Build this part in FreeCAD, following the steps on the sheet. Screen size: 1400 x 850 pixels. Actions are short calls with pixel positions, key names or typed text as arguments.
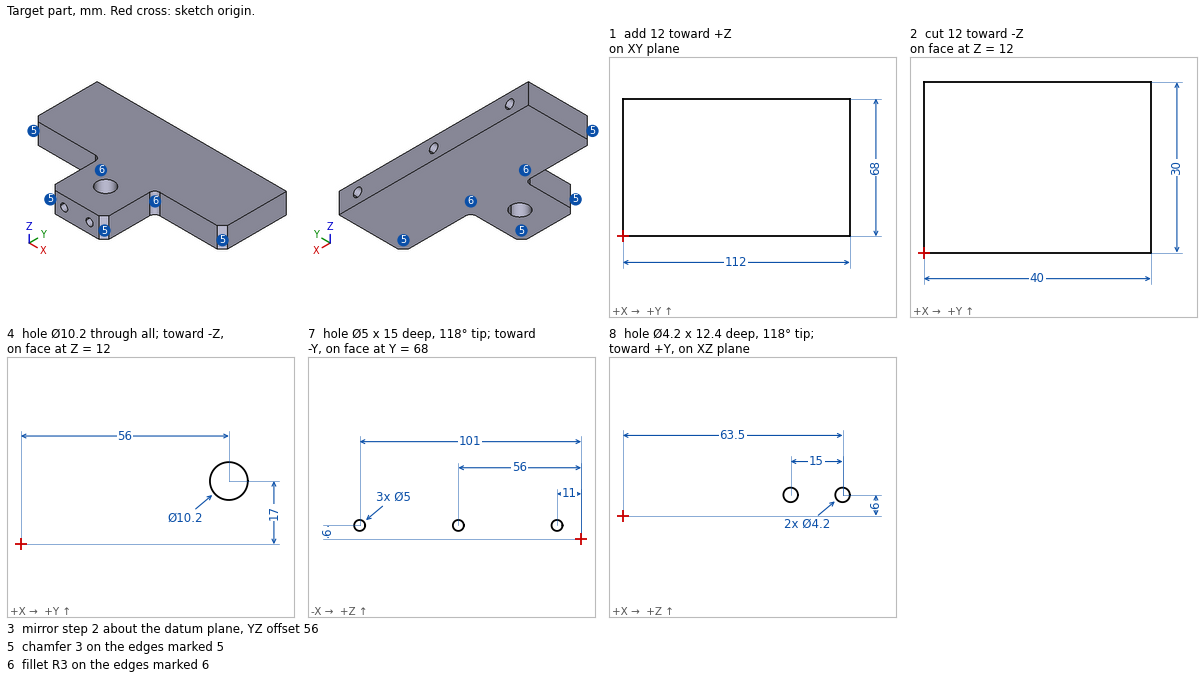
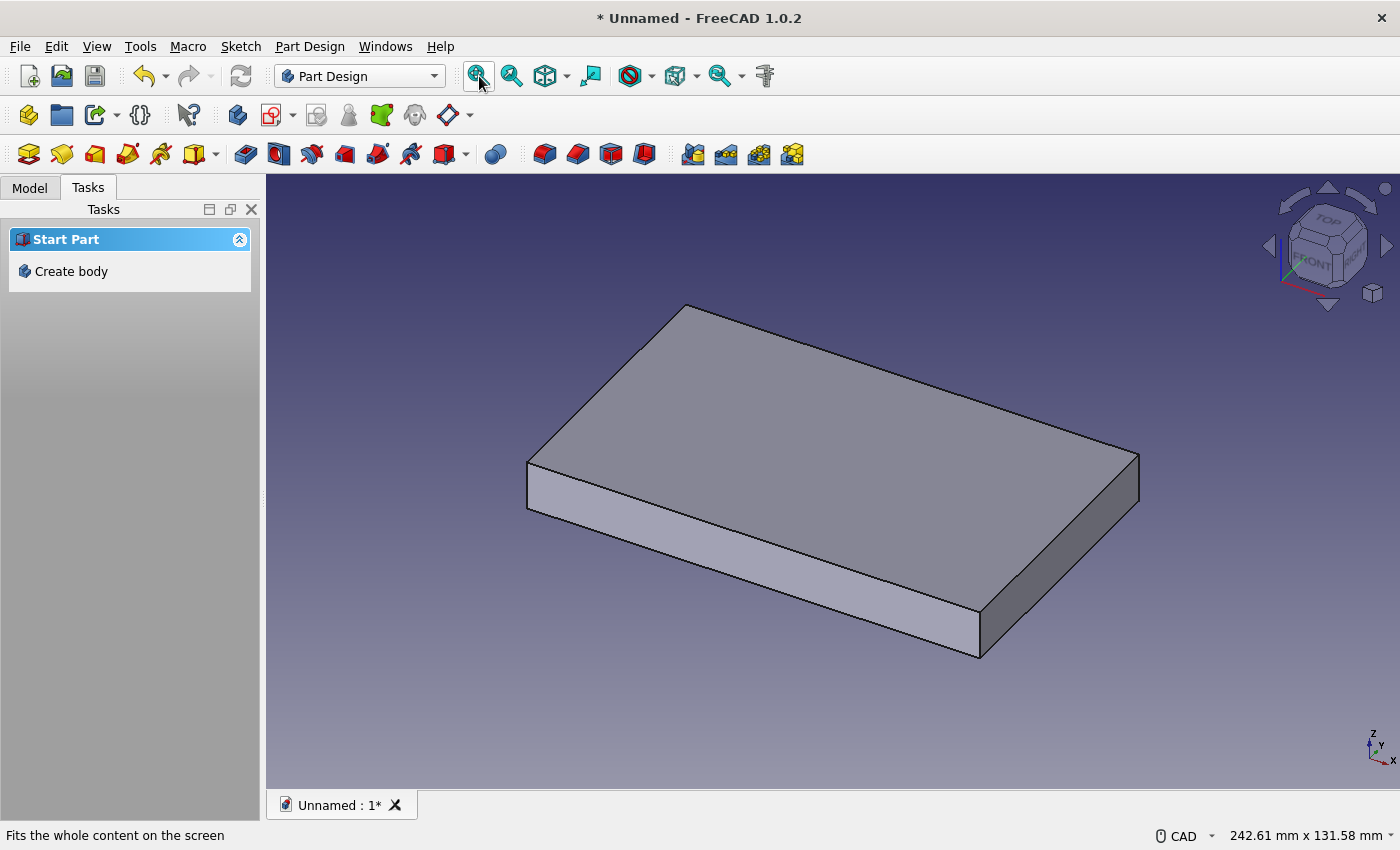
click(898, 479)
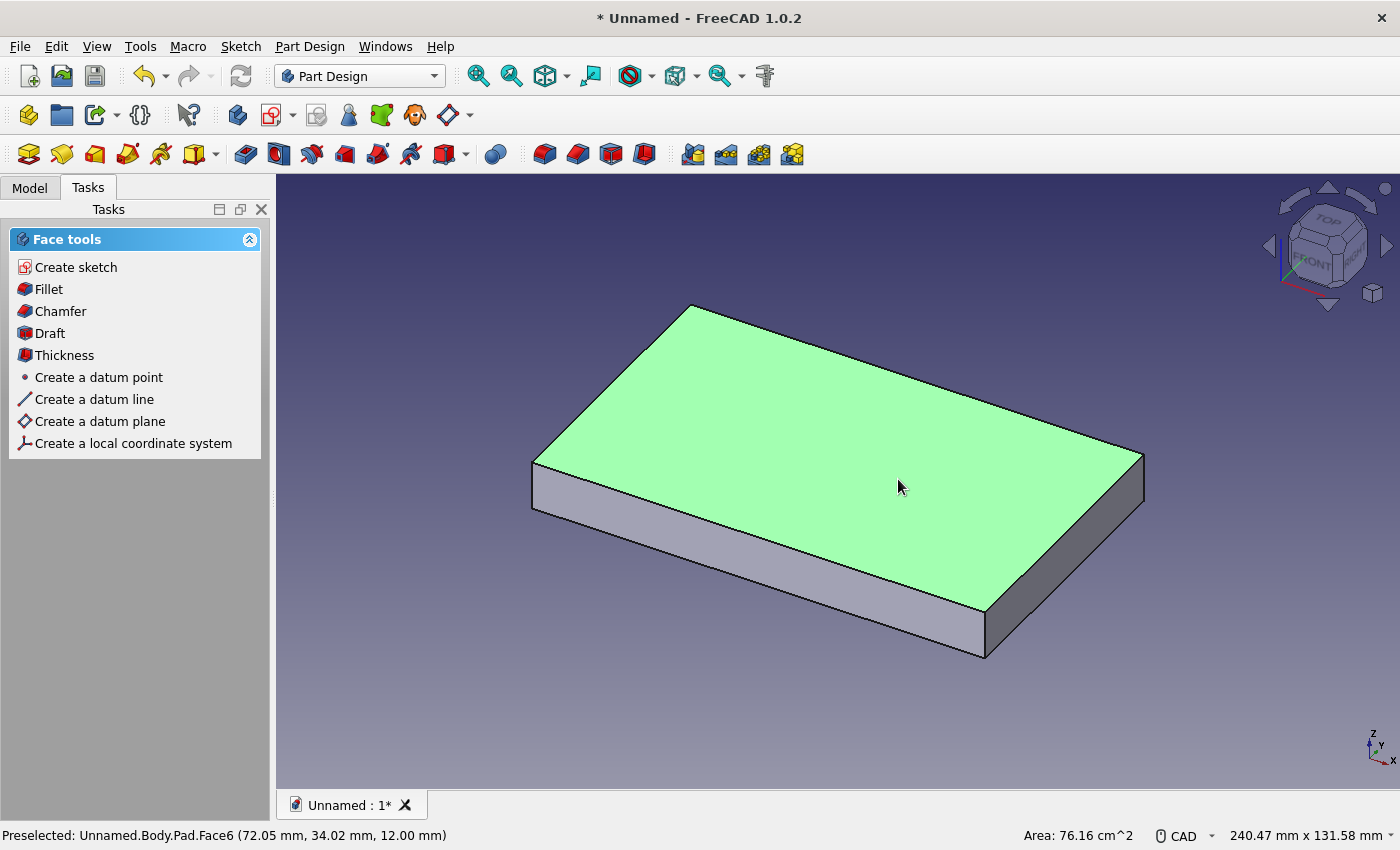
click(270, 116)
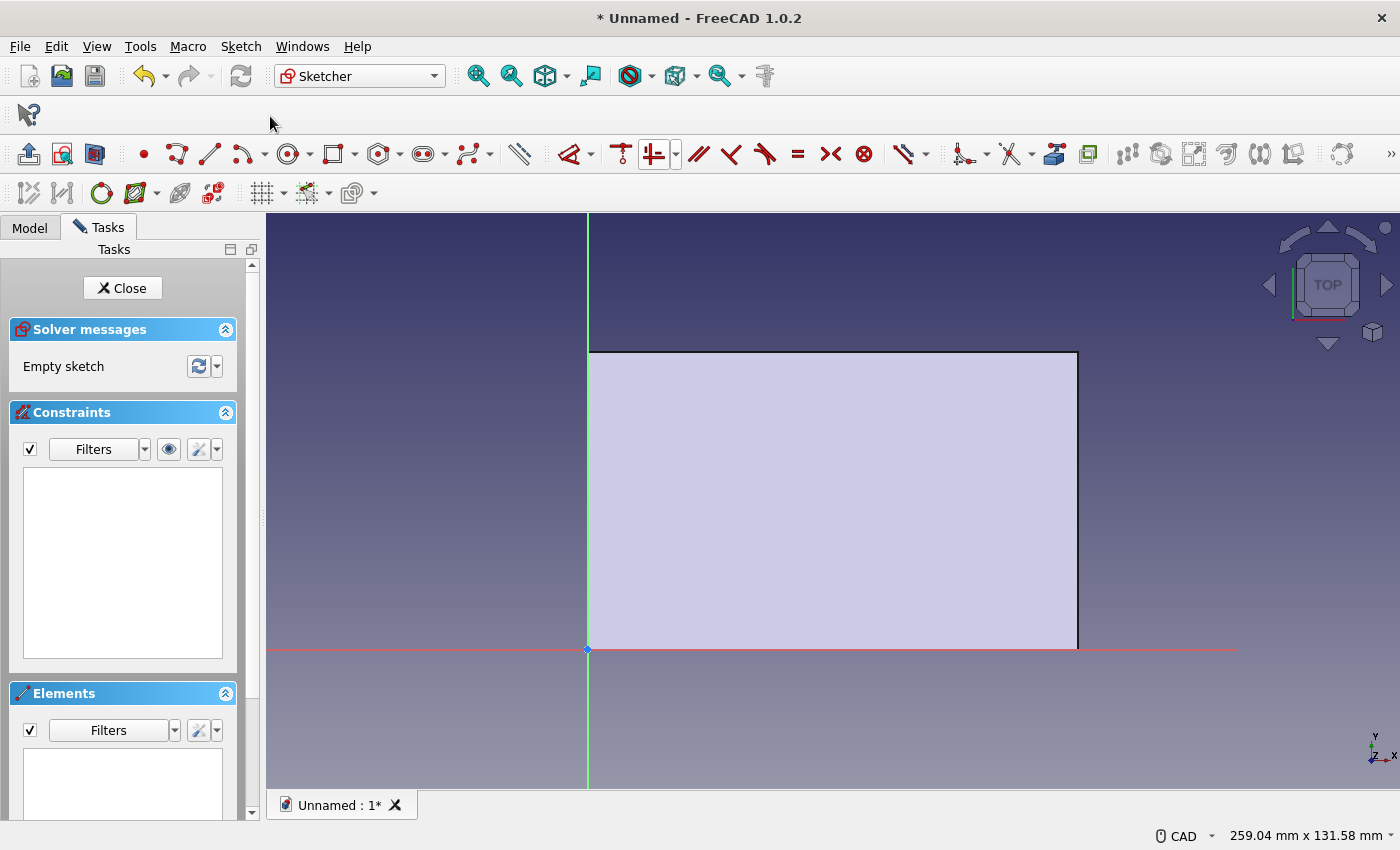
scroll(624, 633, up, 5)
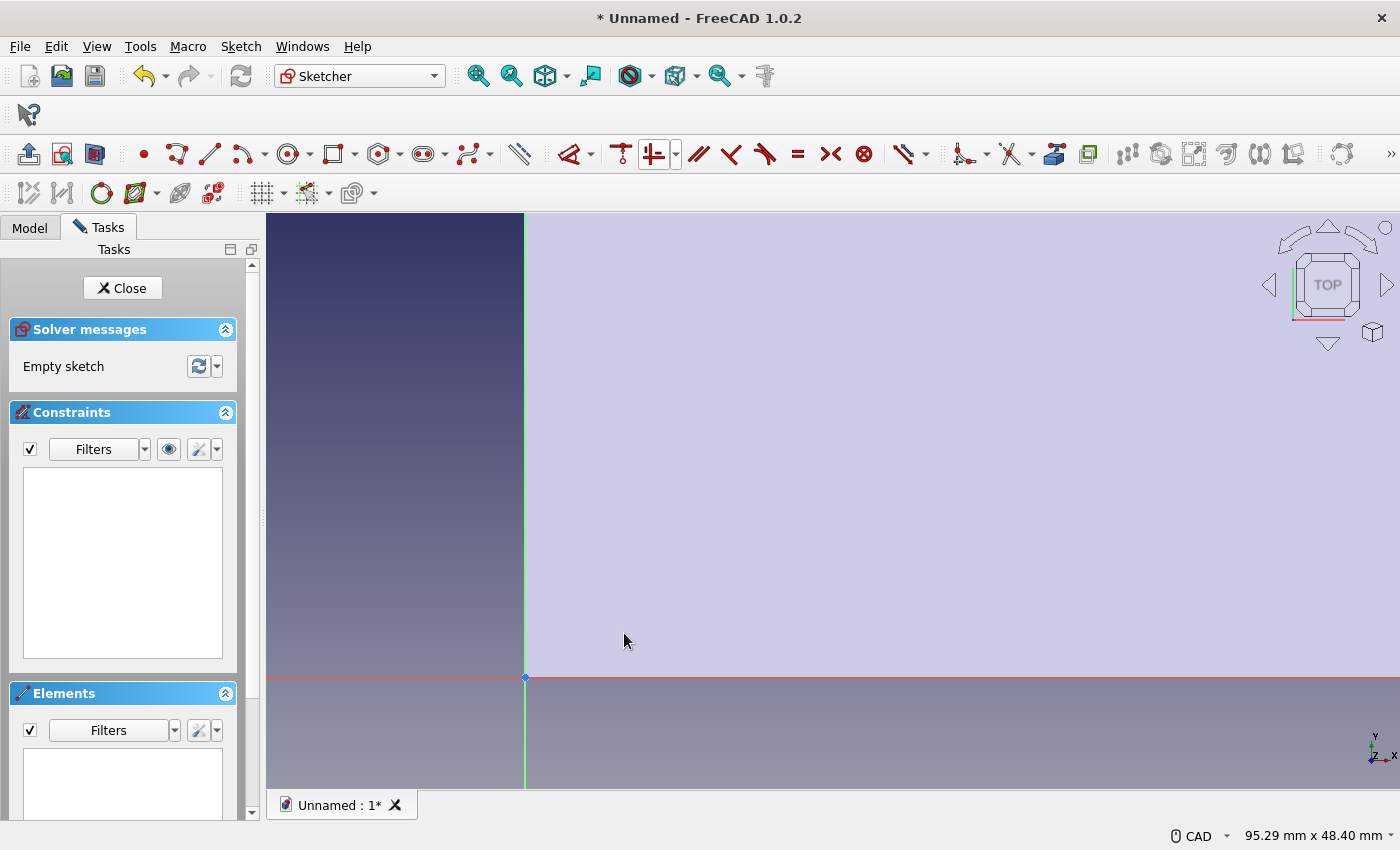
click(332, 154)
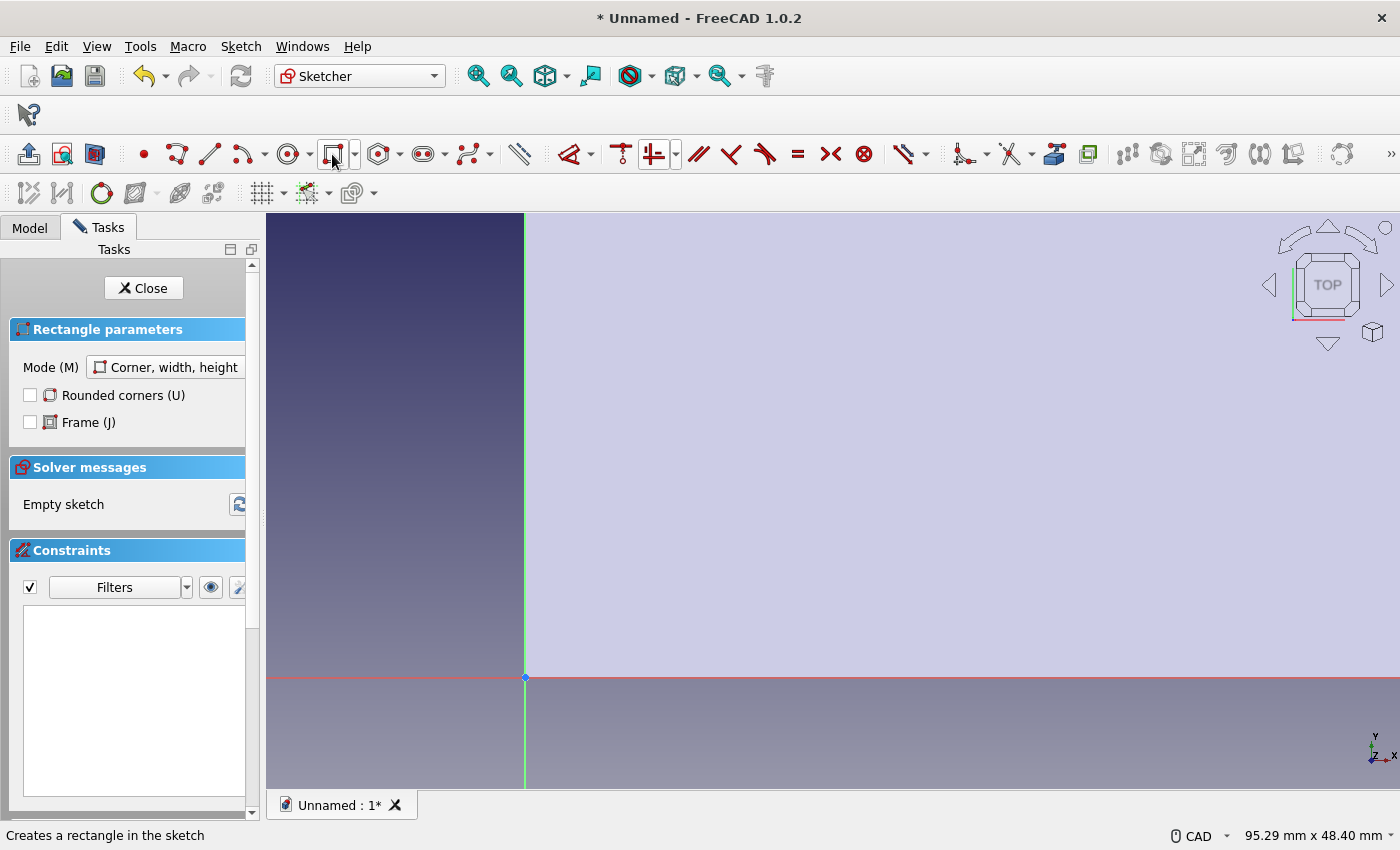
click(525, 678)
click(1001, 321)
key(Escape)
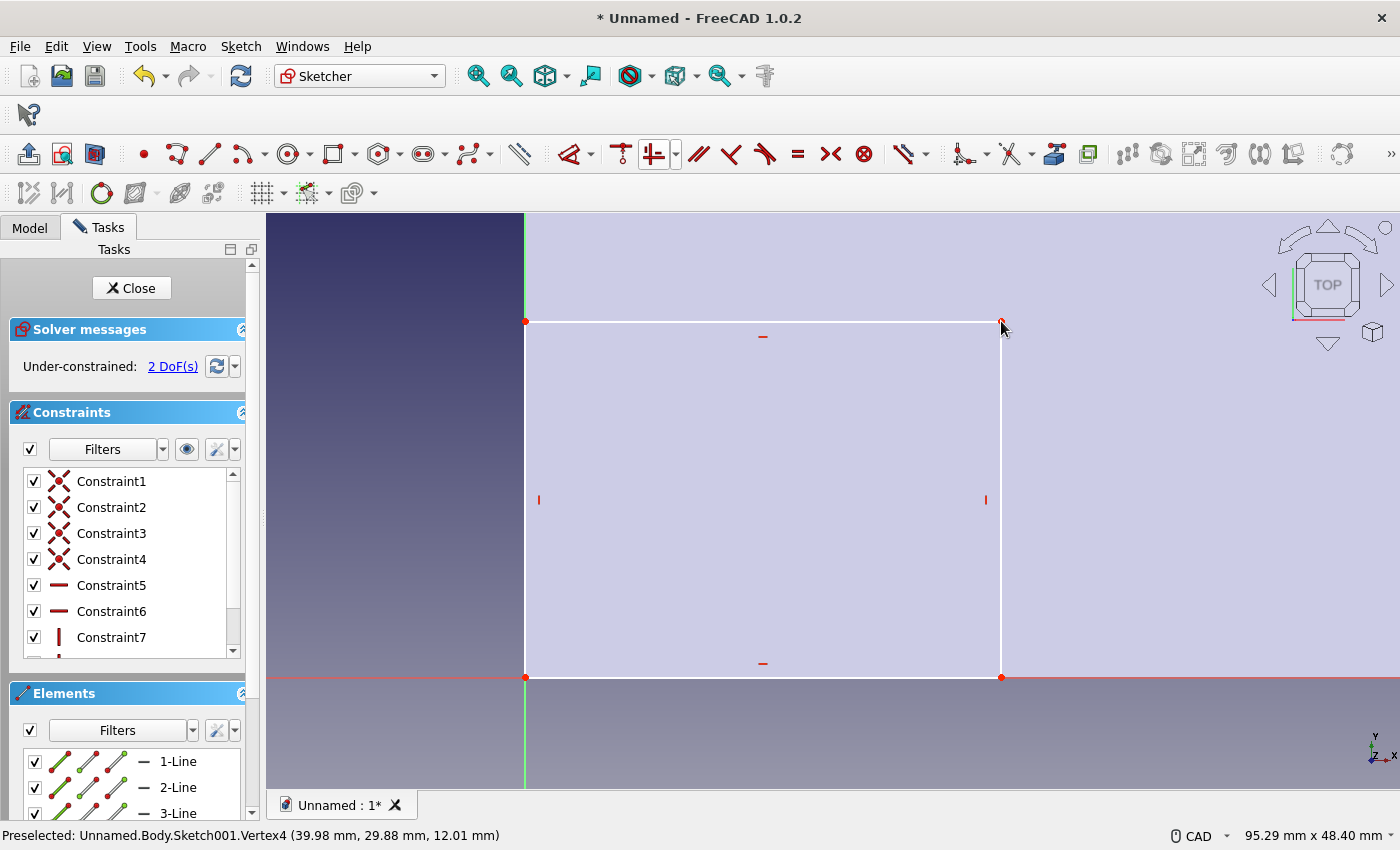
click(568, 154)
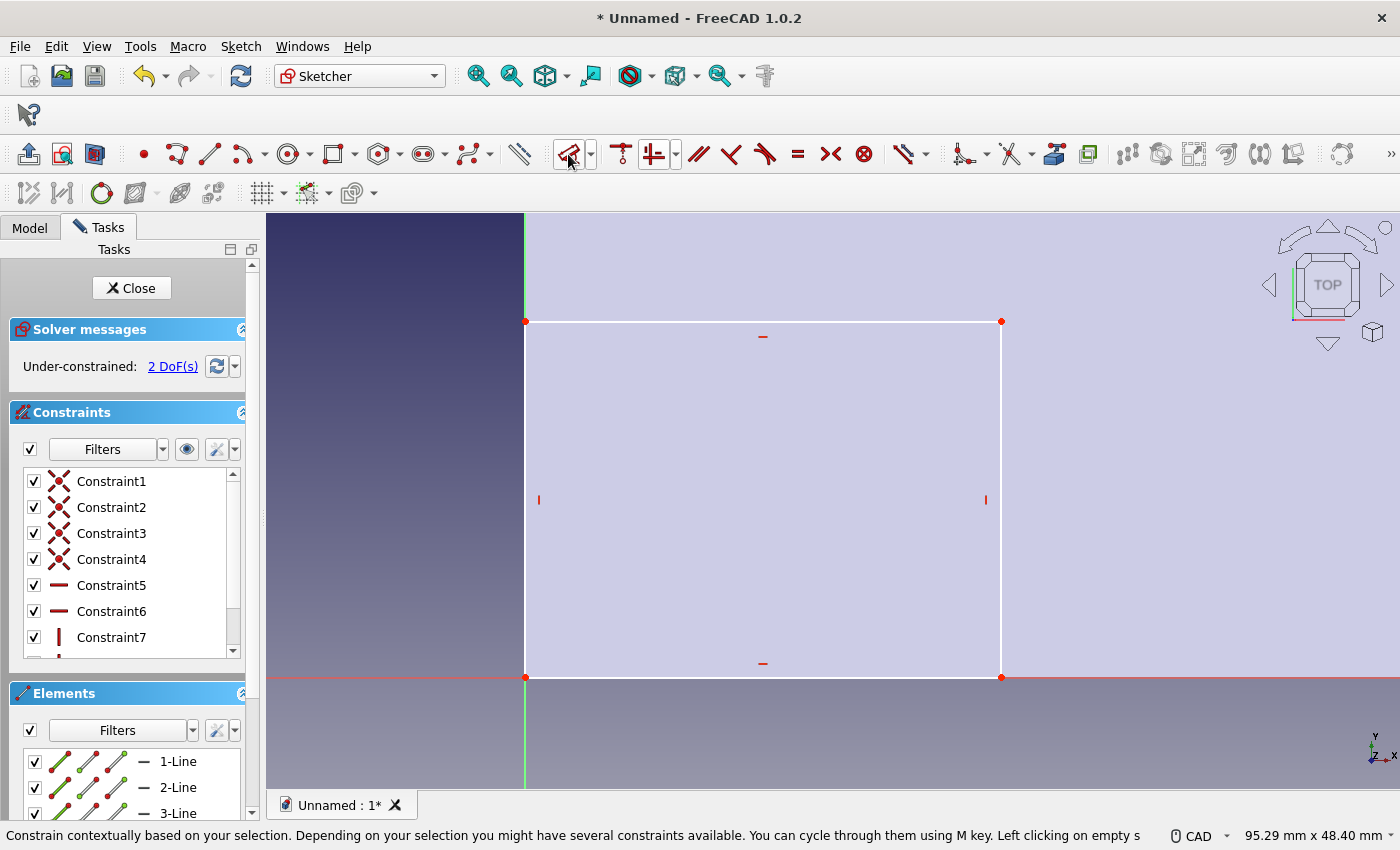
click(668, 678)
click(763, 712)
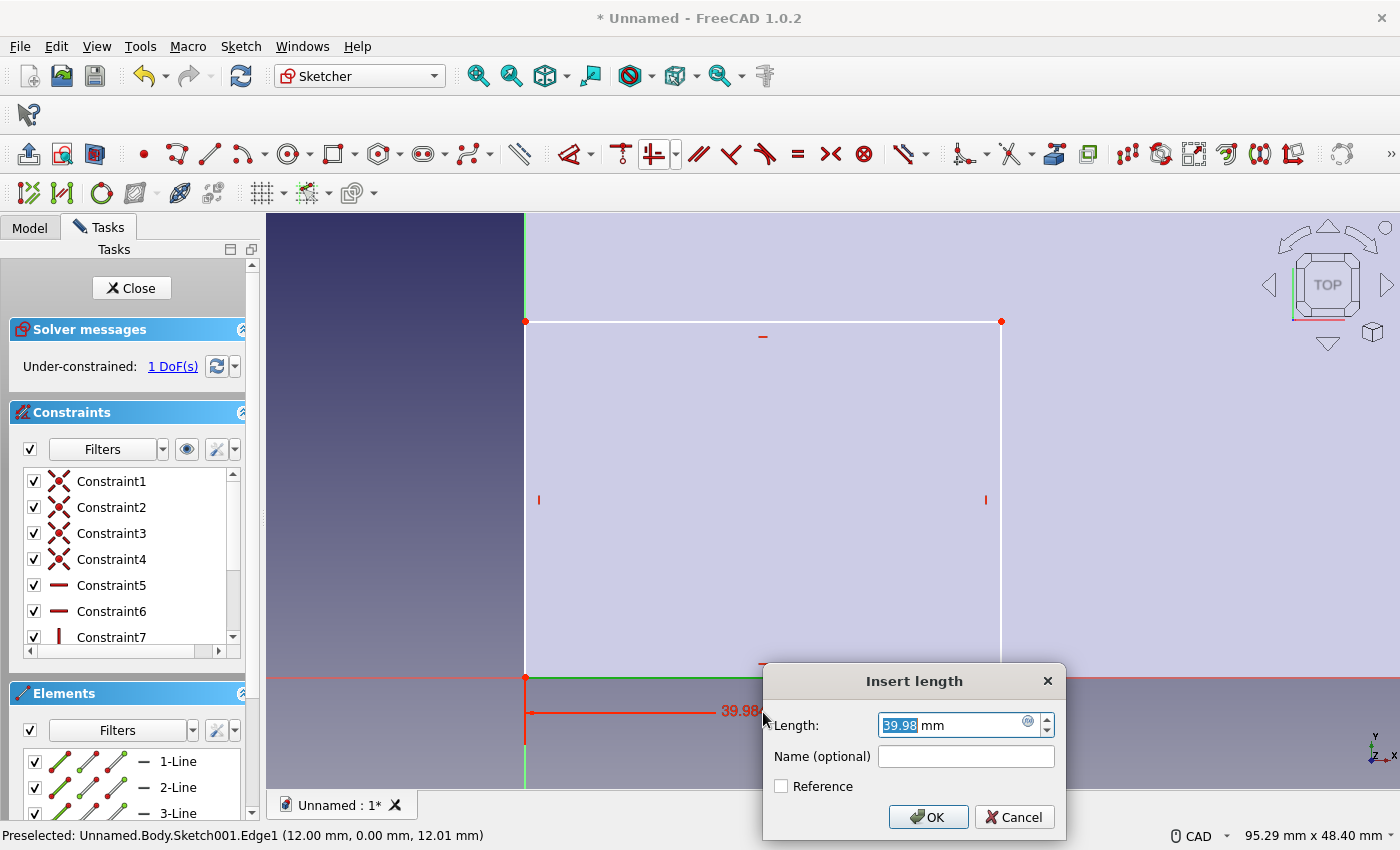
text(40)
key(Return)